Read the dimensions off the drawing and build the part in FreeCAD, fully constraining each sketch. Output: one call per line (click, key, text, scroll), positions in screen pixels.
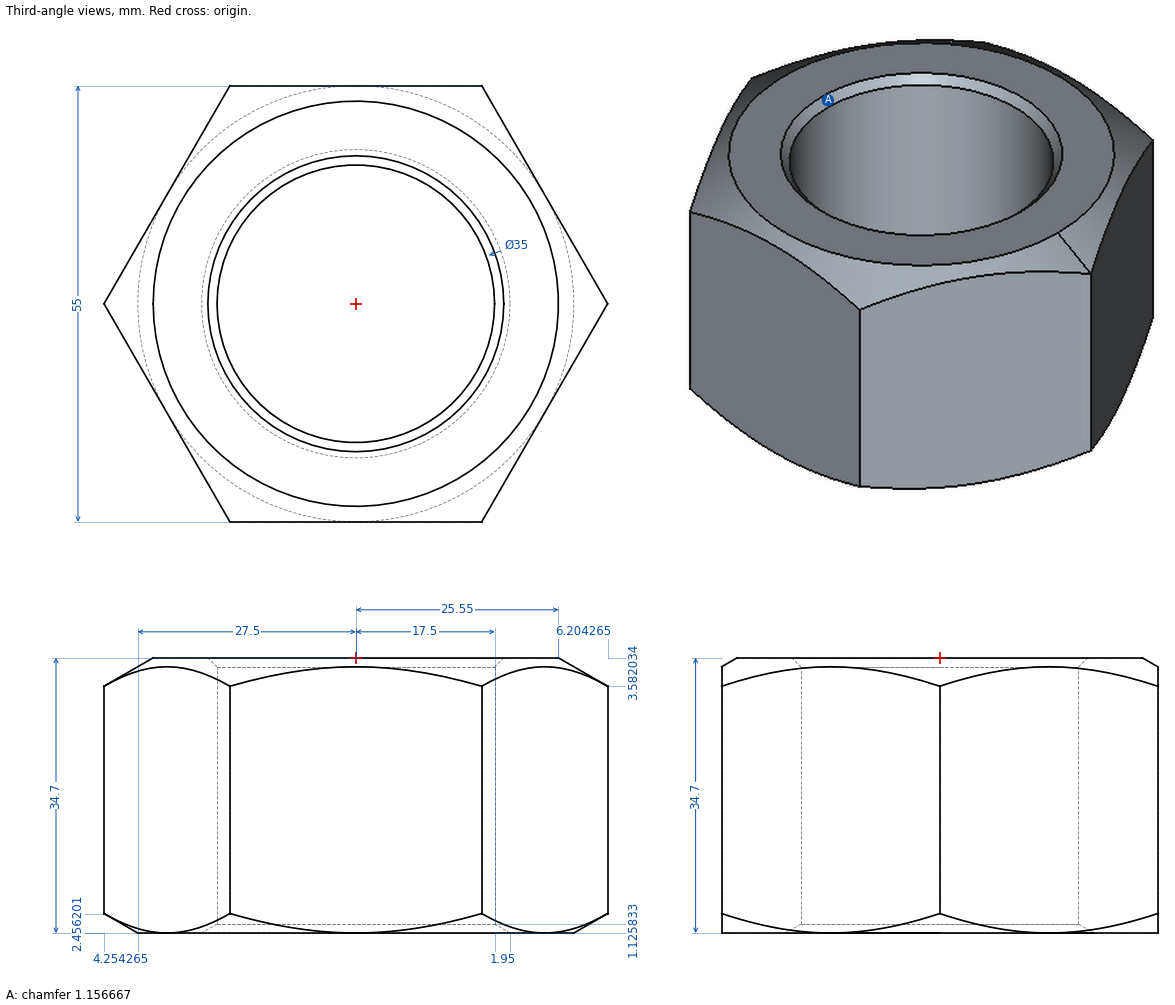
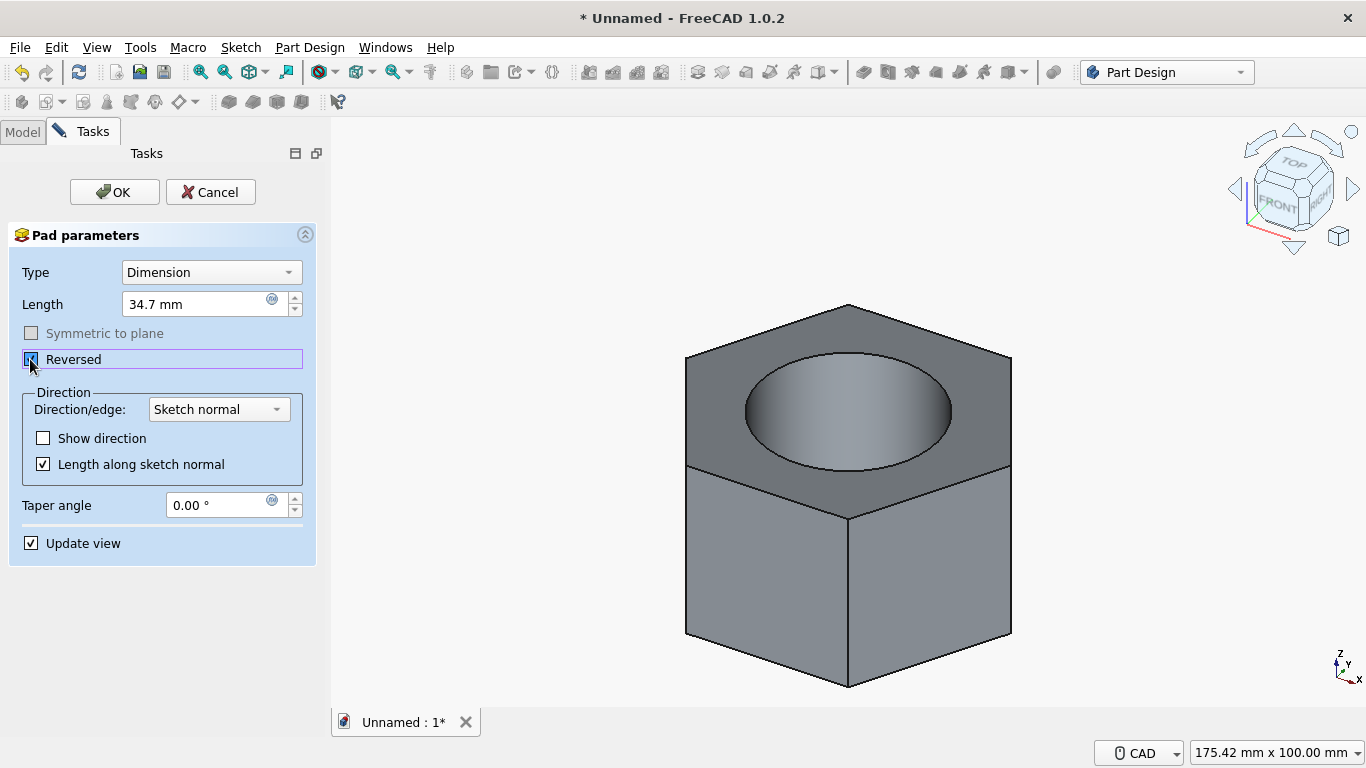
click(115, 192)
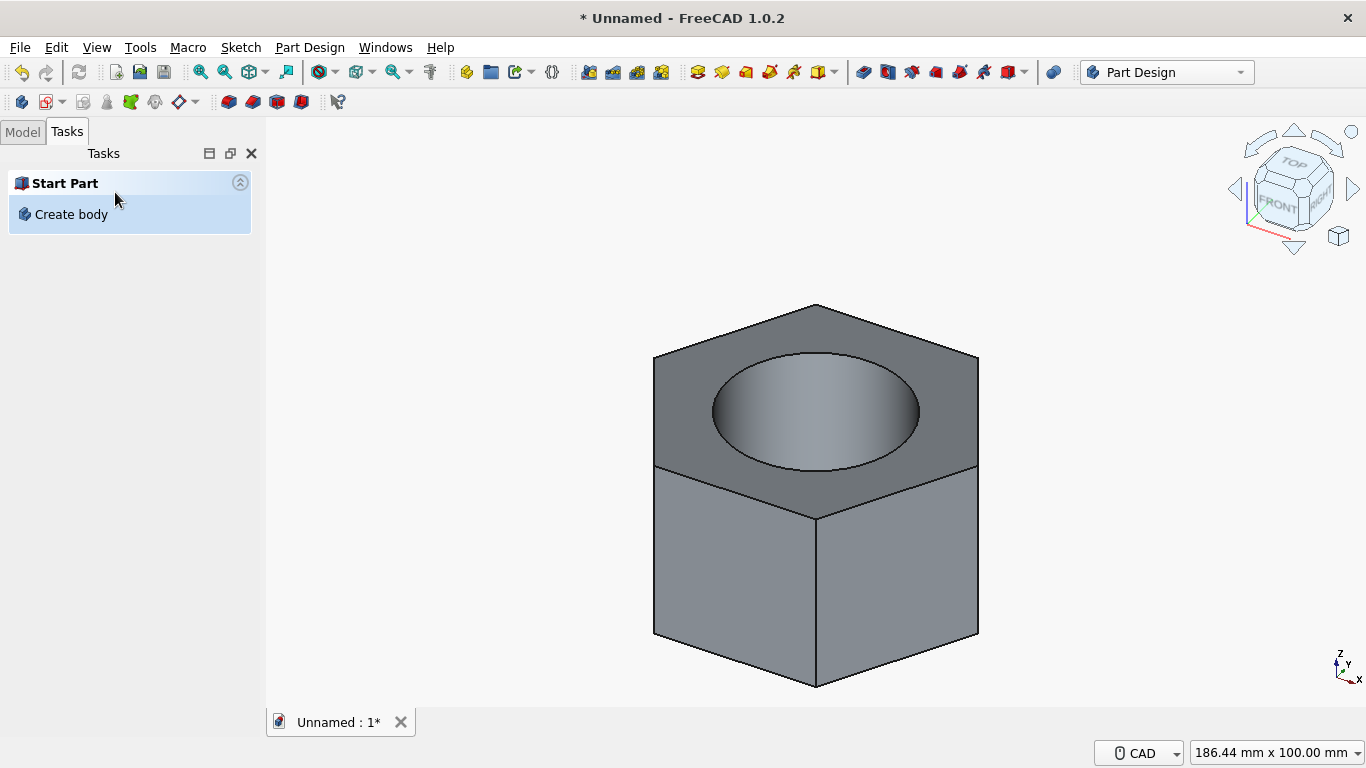
key(v)
key(f)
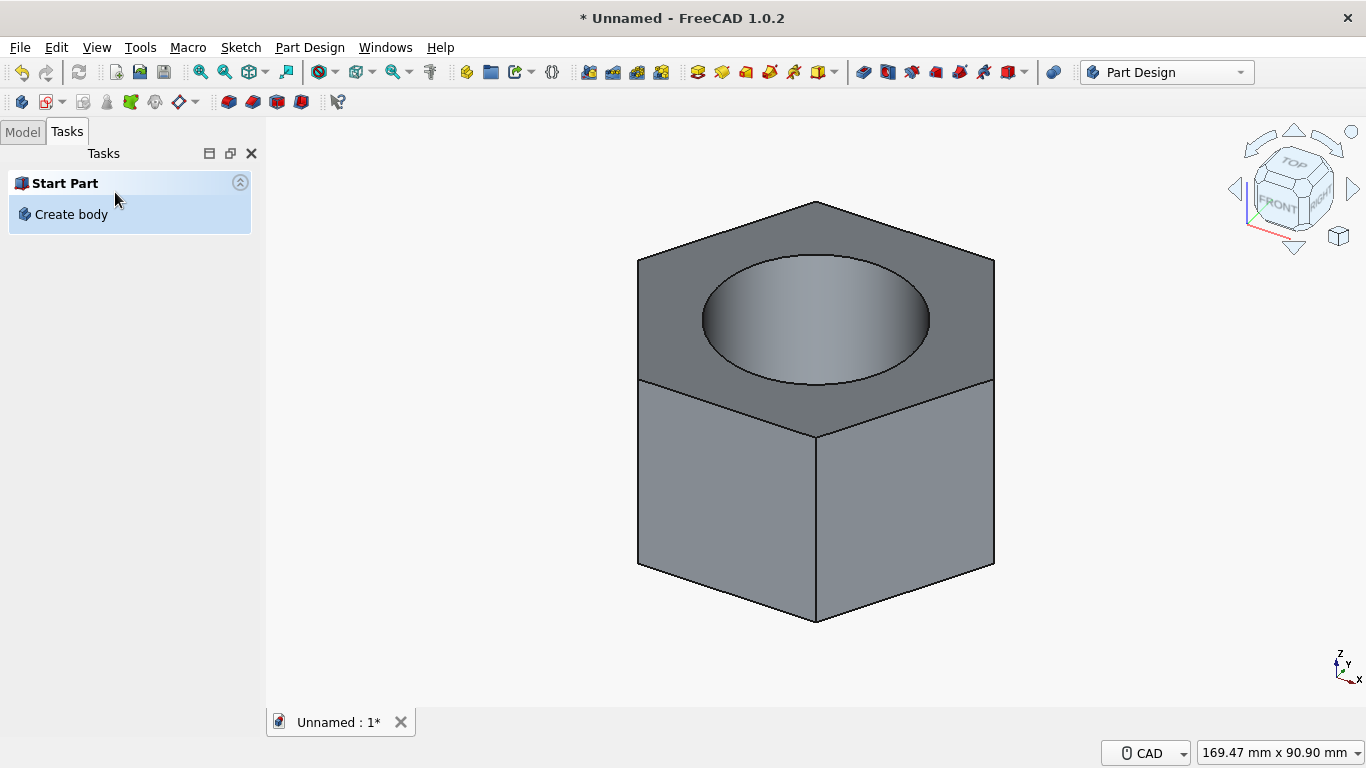
click(46, 102)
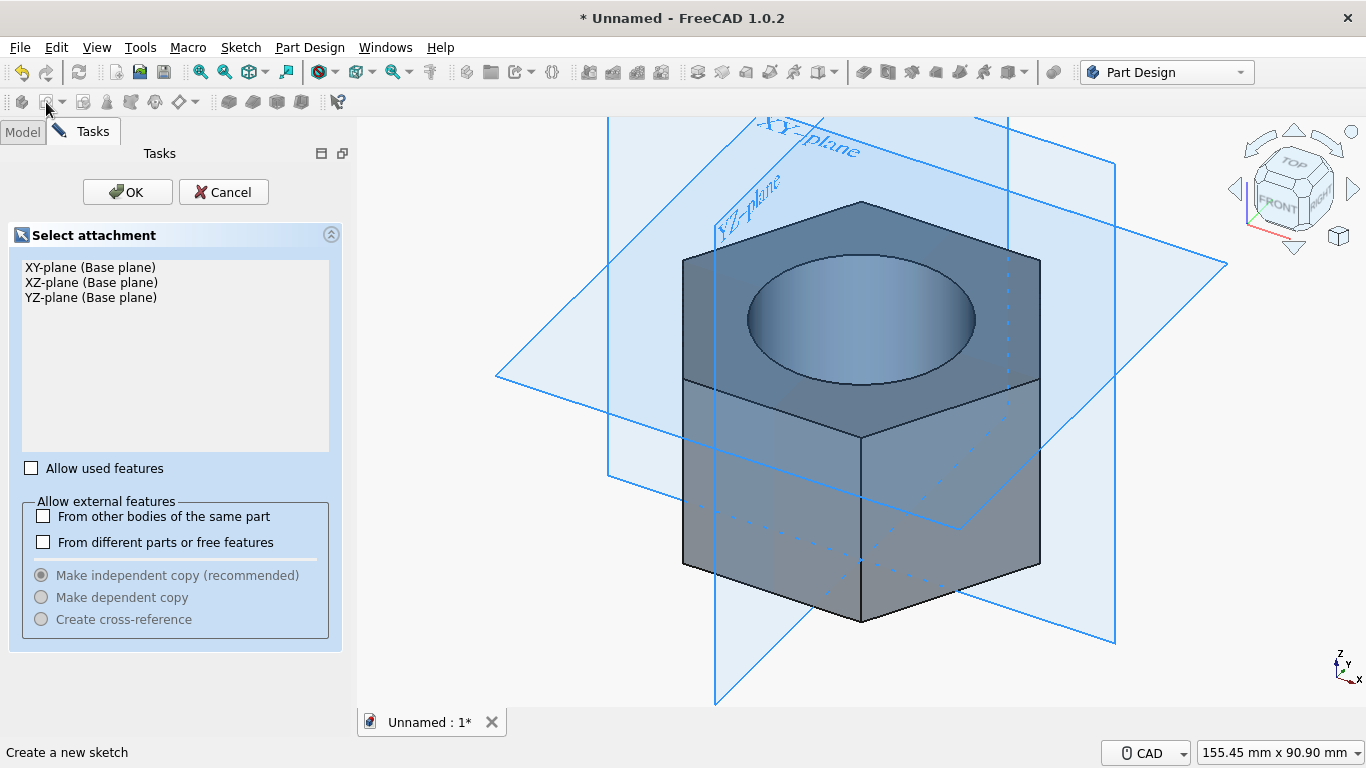
click(82, 282)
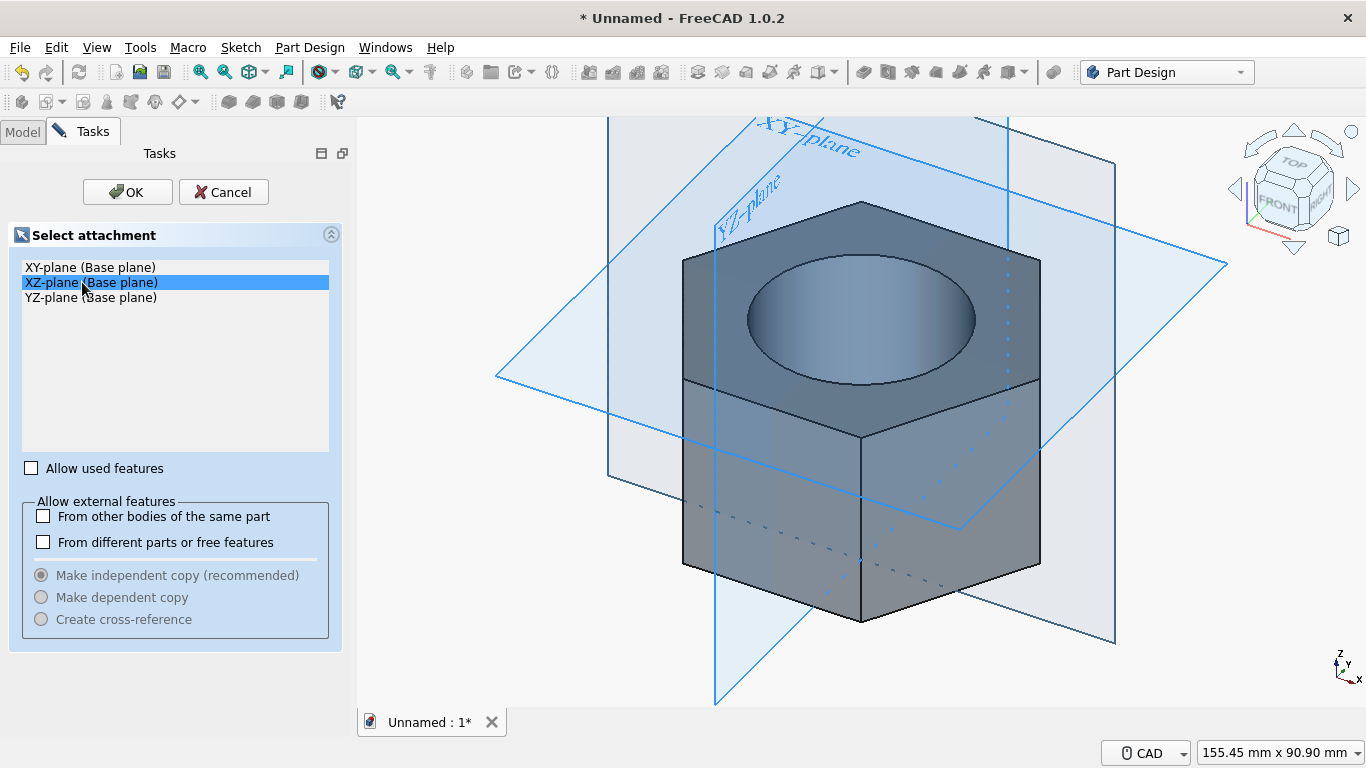
click(128, 192)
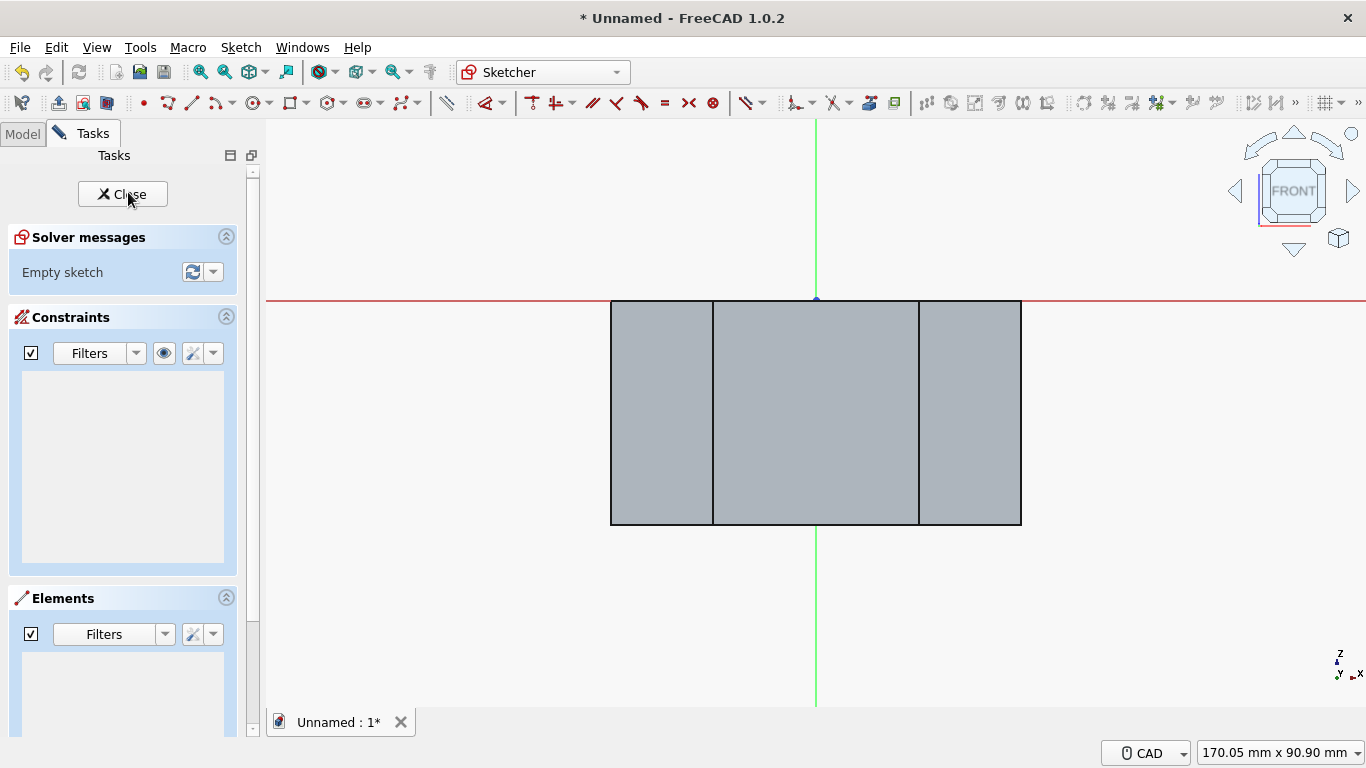
click(108, 104)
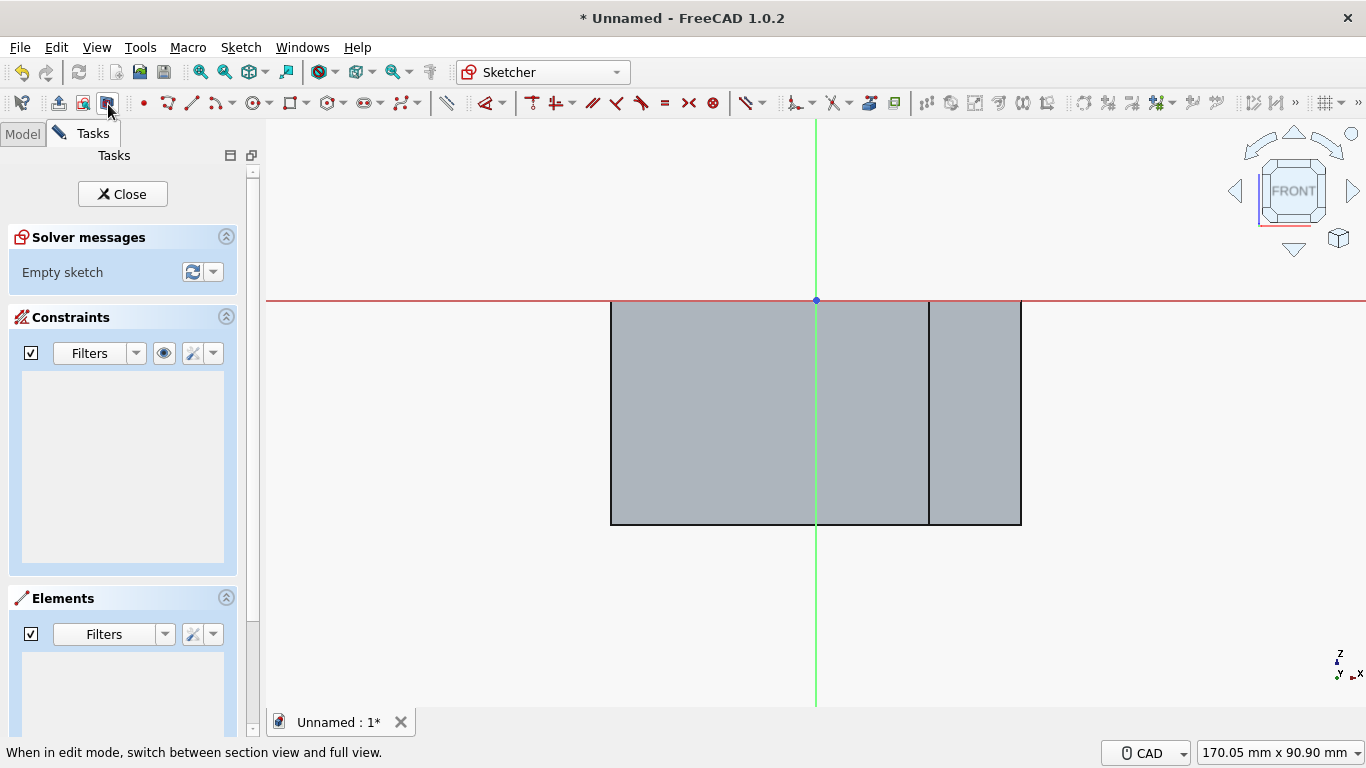
scroll(618, 523, up, 15)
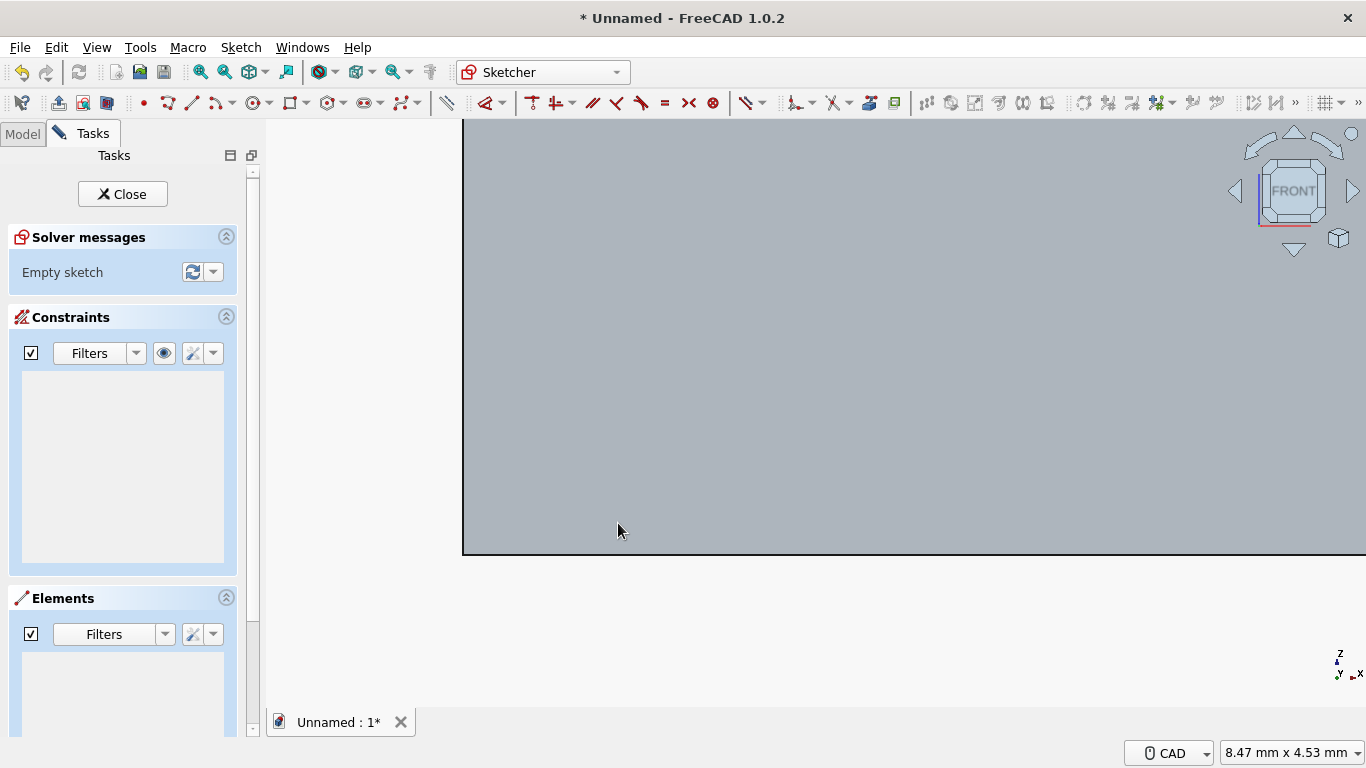
click(168, 104)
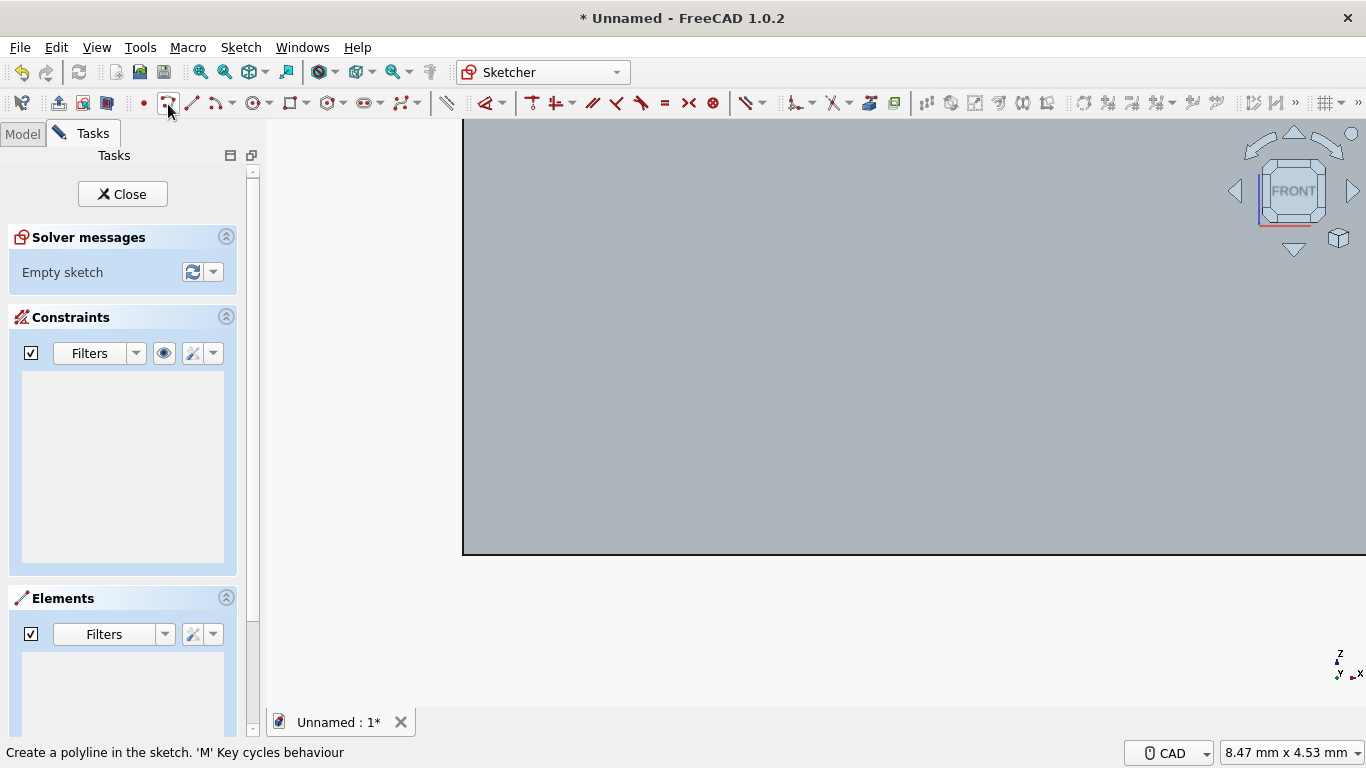
click(1016, 555)
click(463, 555)
click(463, 236)
click(1016, 556)
key(Escape)
key(Escape)